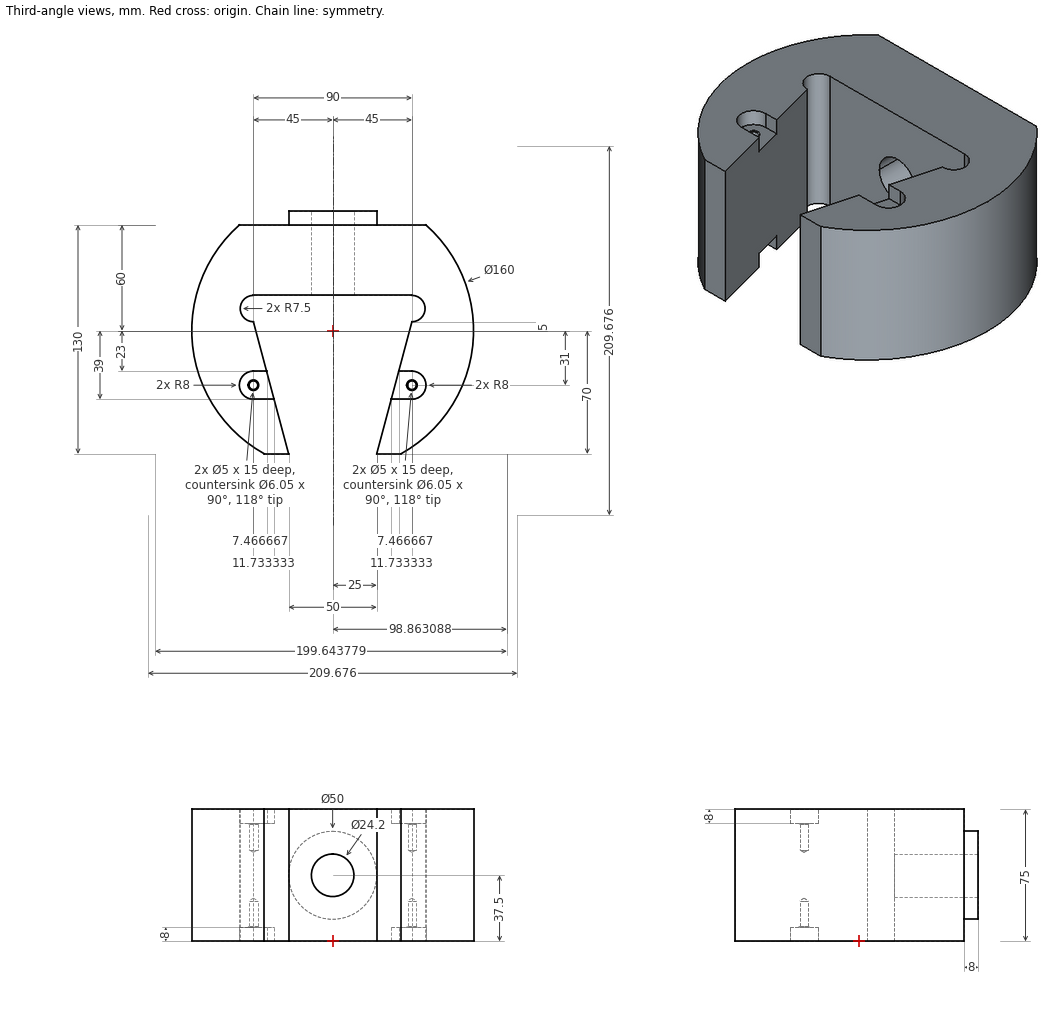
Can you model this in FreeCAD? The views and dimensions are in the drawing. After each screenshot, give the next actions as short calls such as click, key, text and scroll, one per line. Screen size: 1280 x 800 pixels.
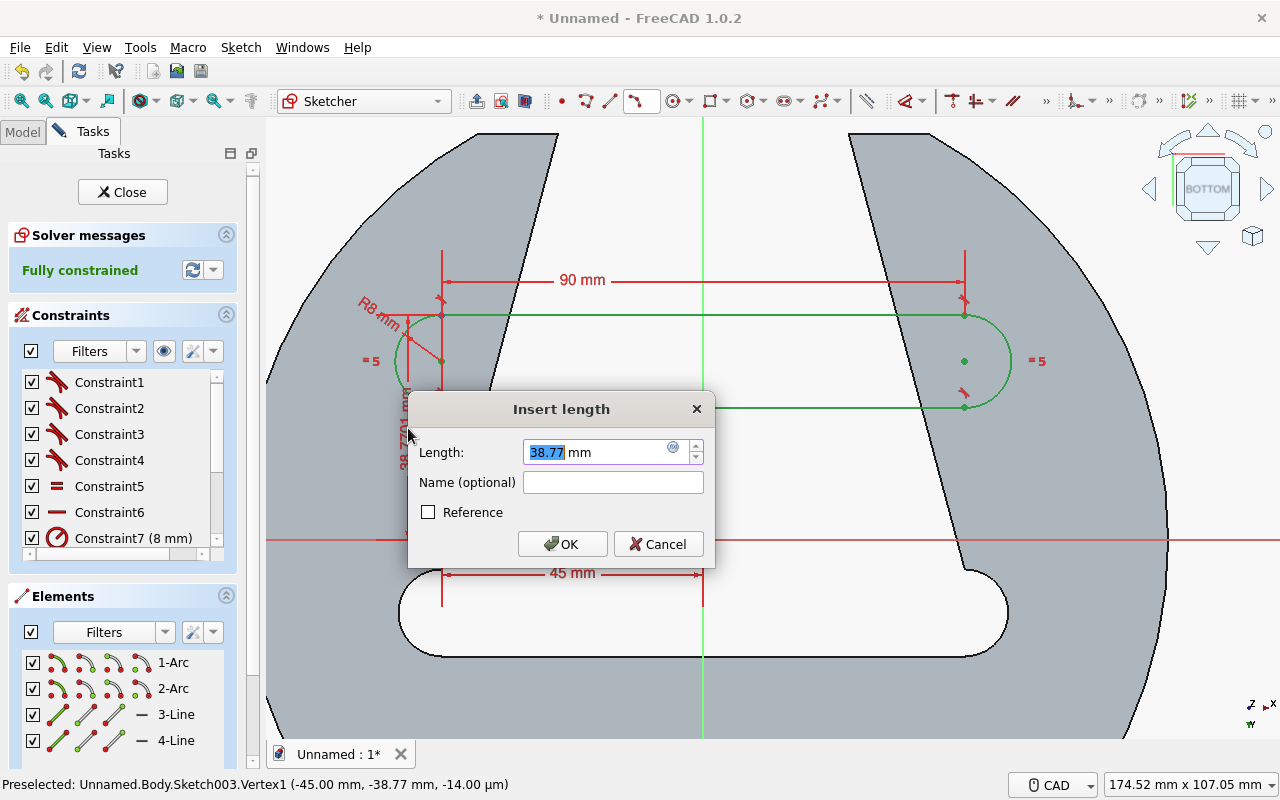
text(39)
key(Return)
key(Escape)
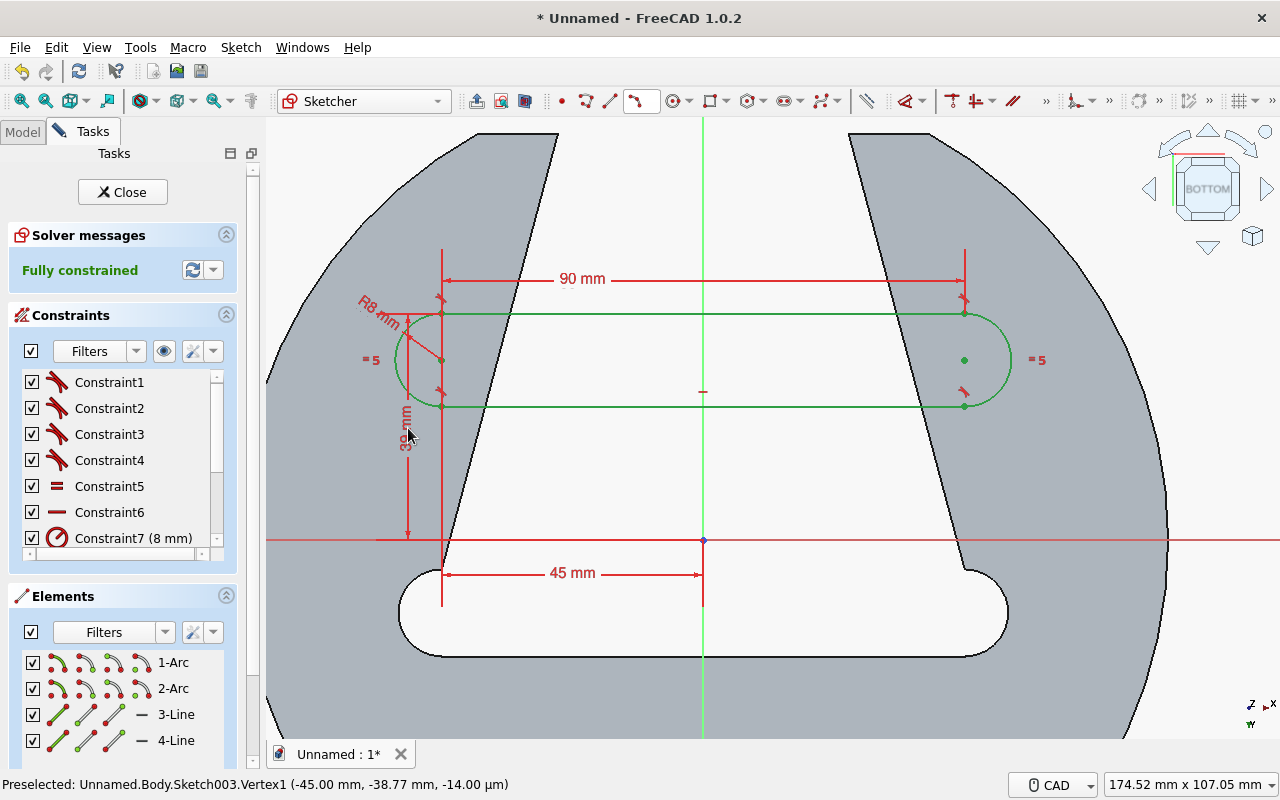
click(123, 192)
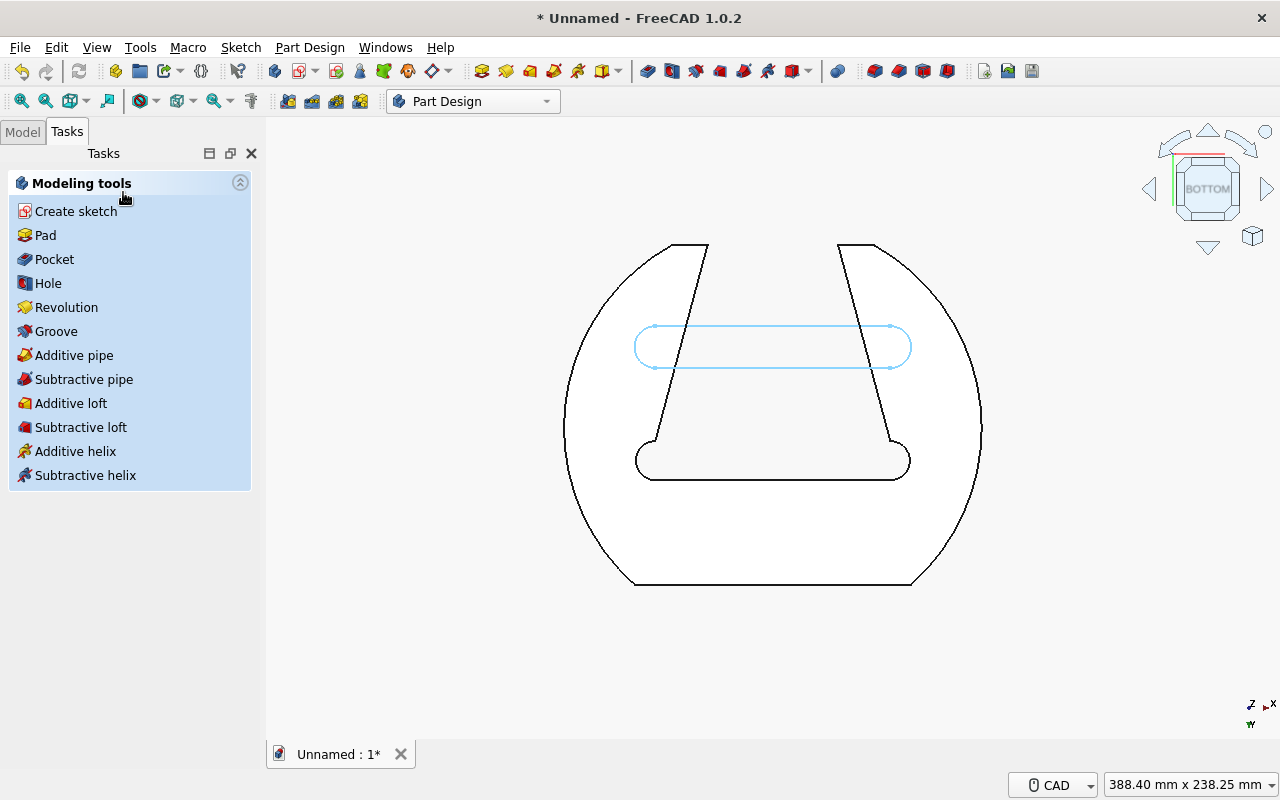
click(648, 72)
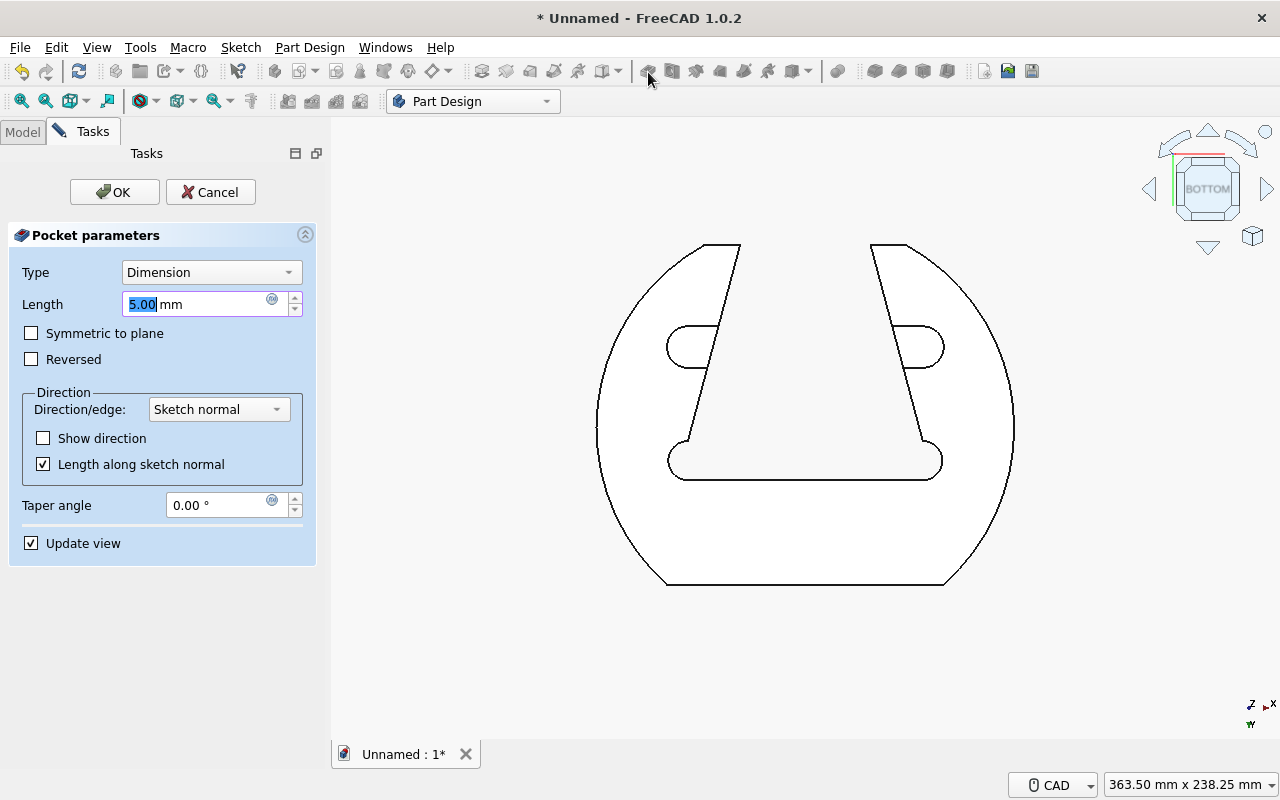
text(8)
key(Tab)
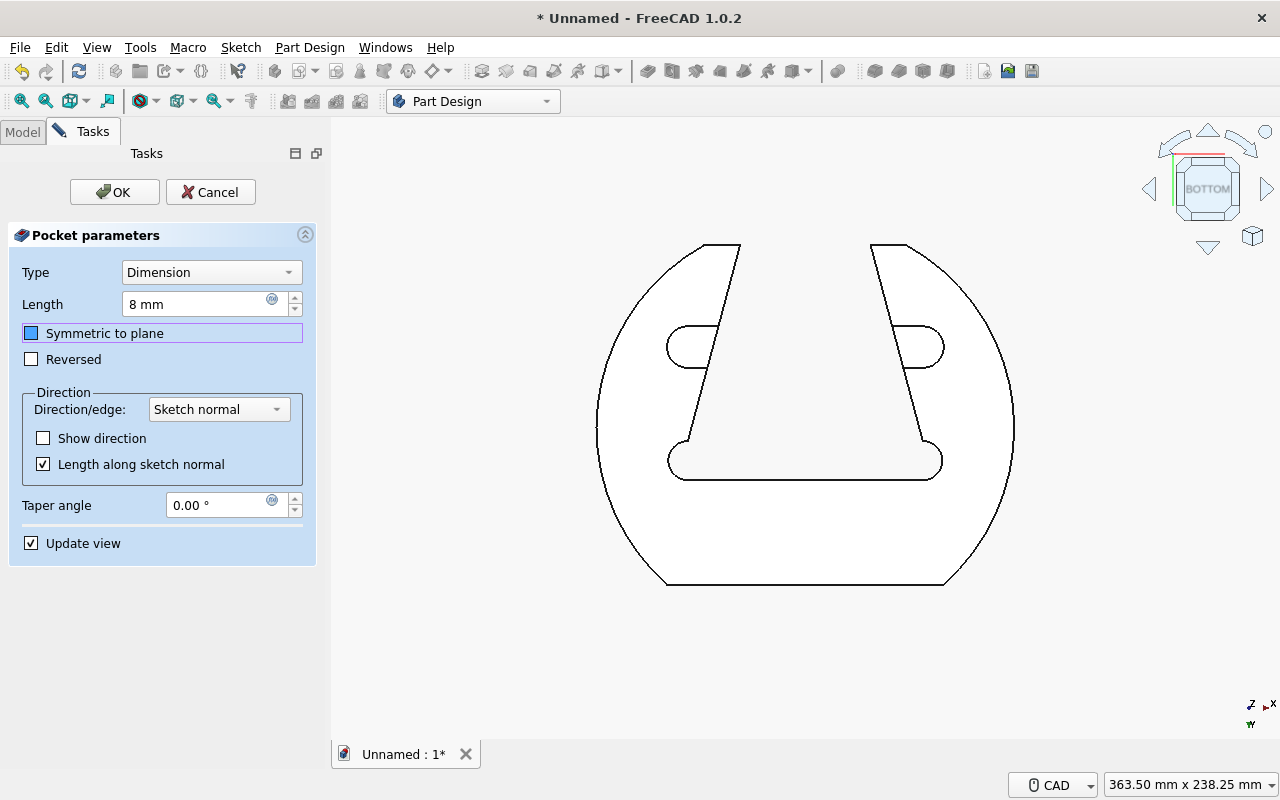
click(115, 192)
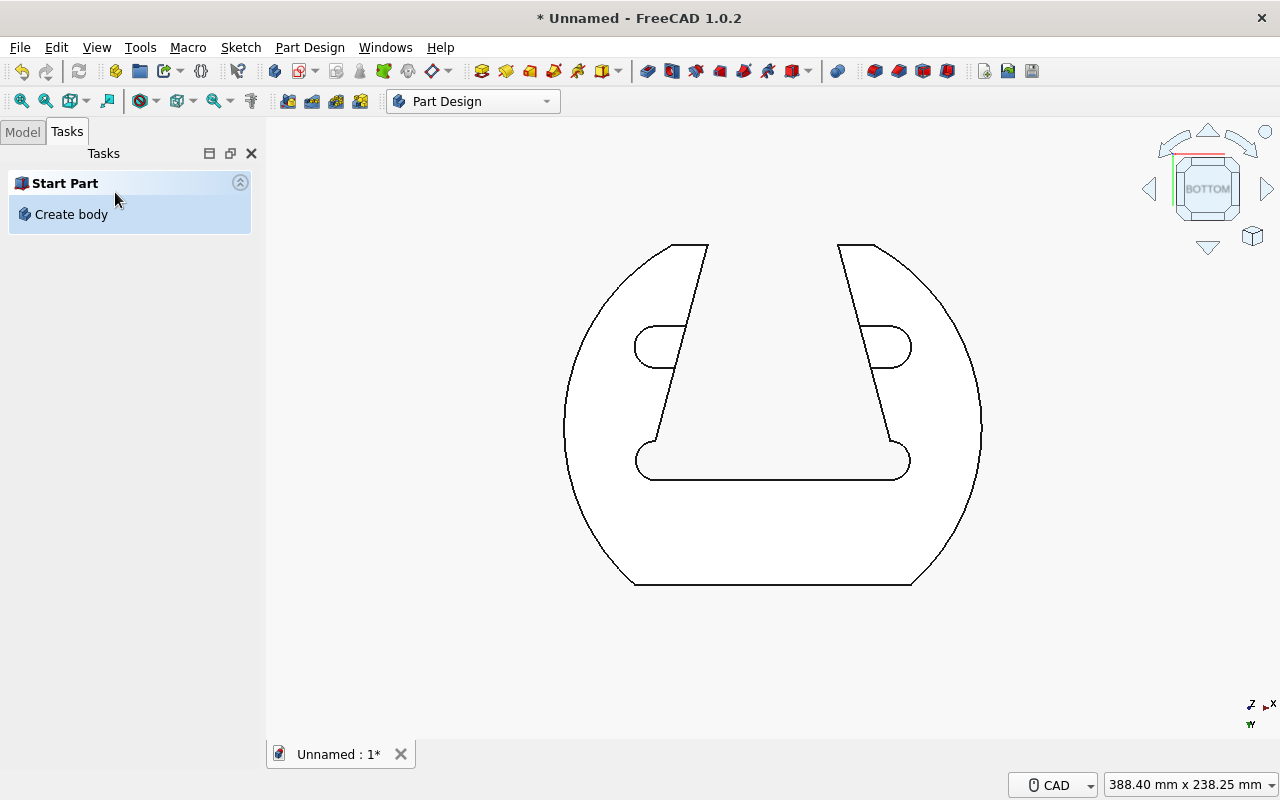
click(23, 131)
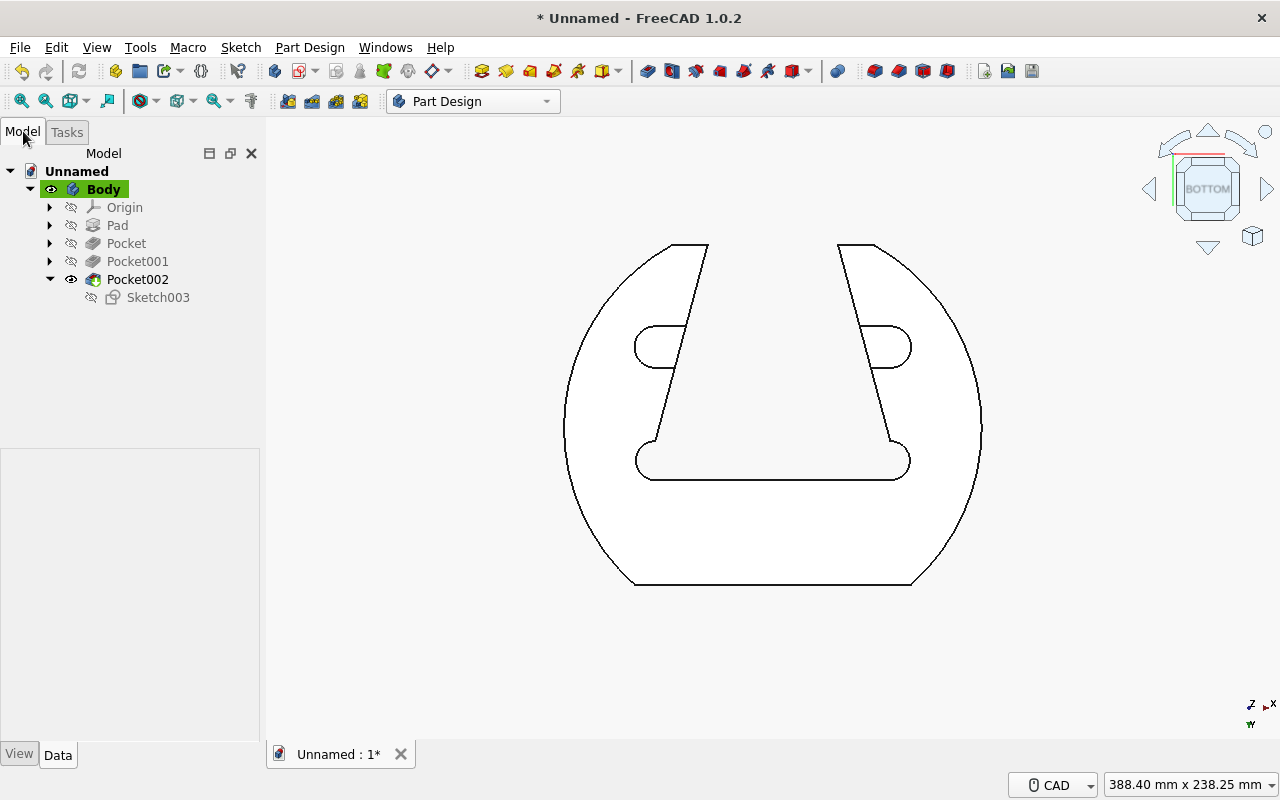
click(50, 207)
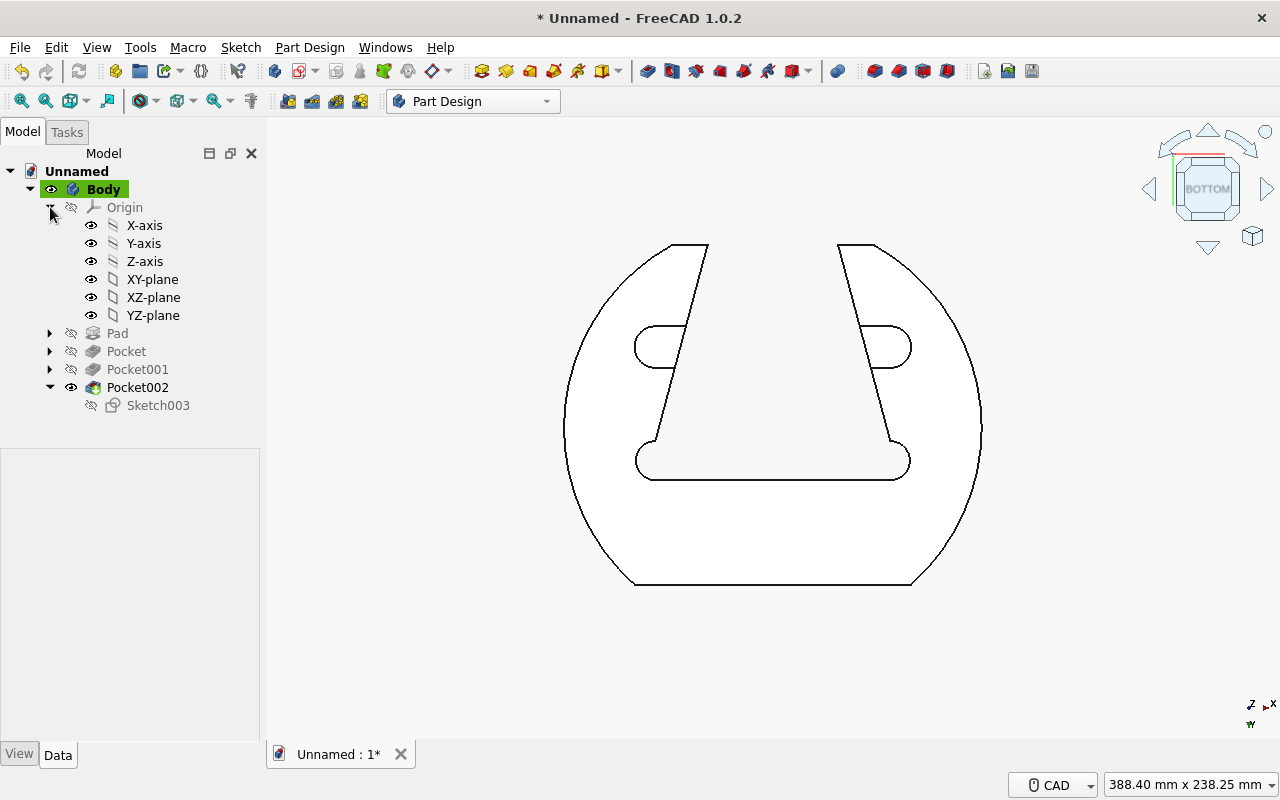
click(136, 279)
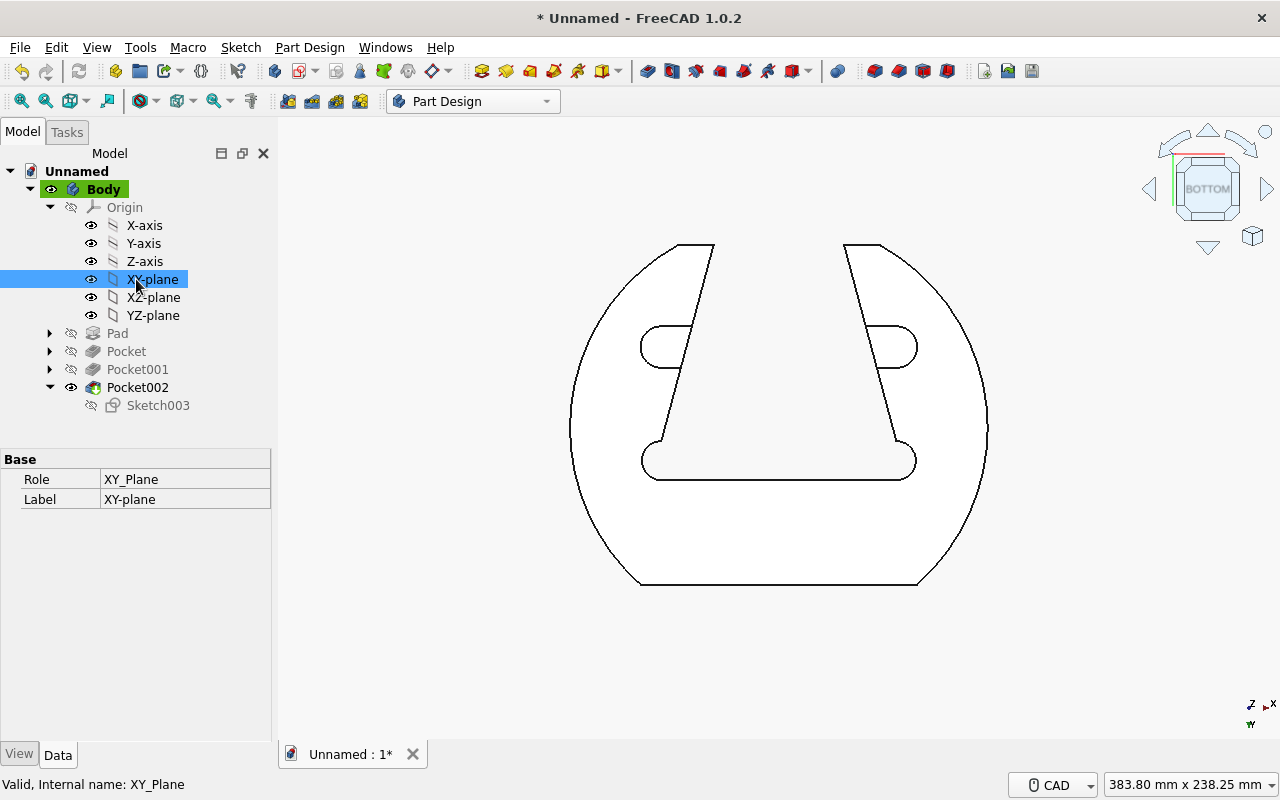
click(432, 72)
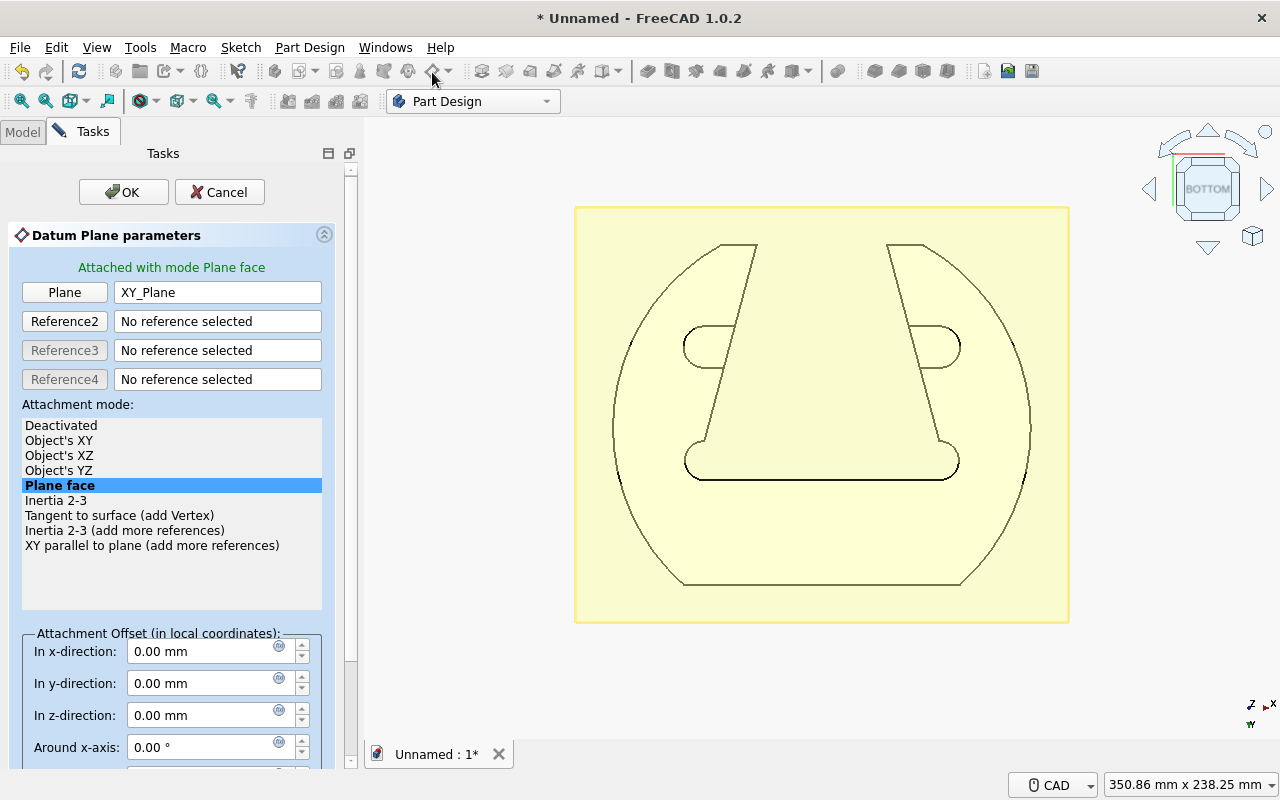
triple_click(210, 715)